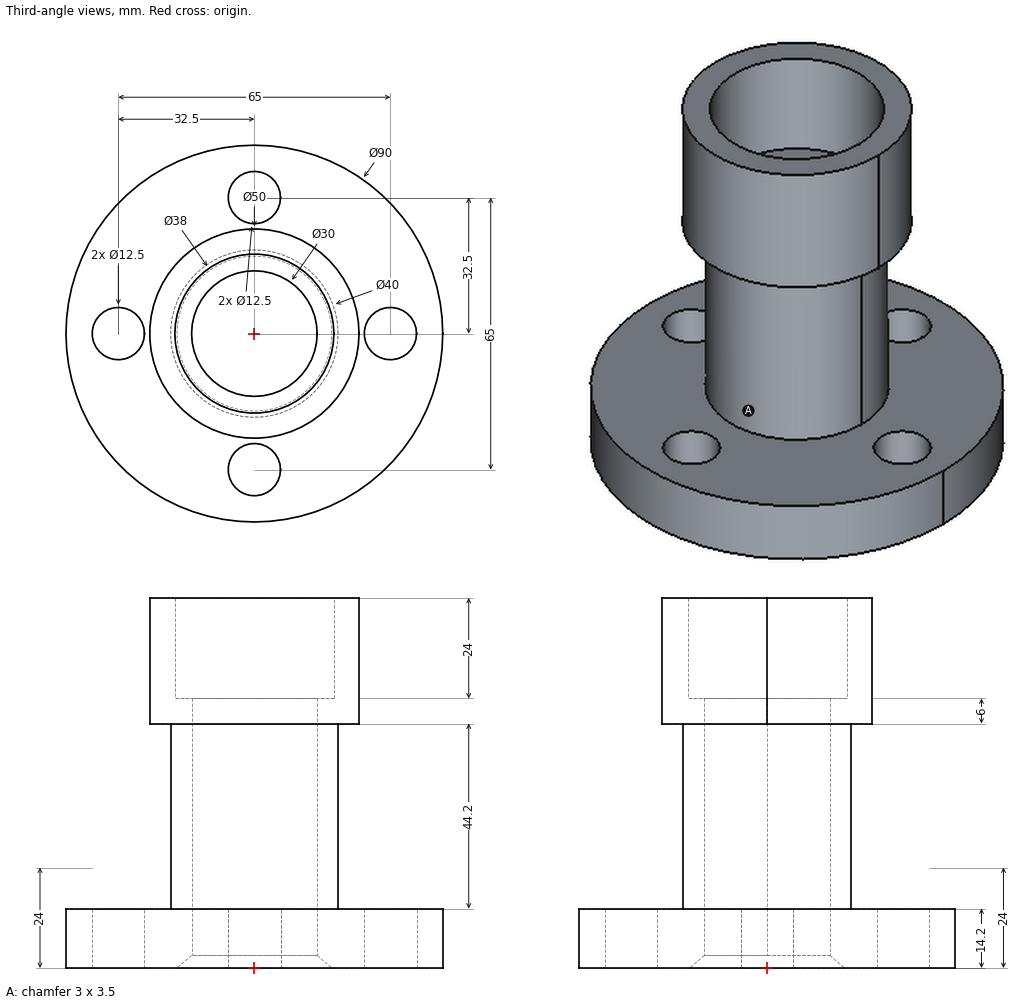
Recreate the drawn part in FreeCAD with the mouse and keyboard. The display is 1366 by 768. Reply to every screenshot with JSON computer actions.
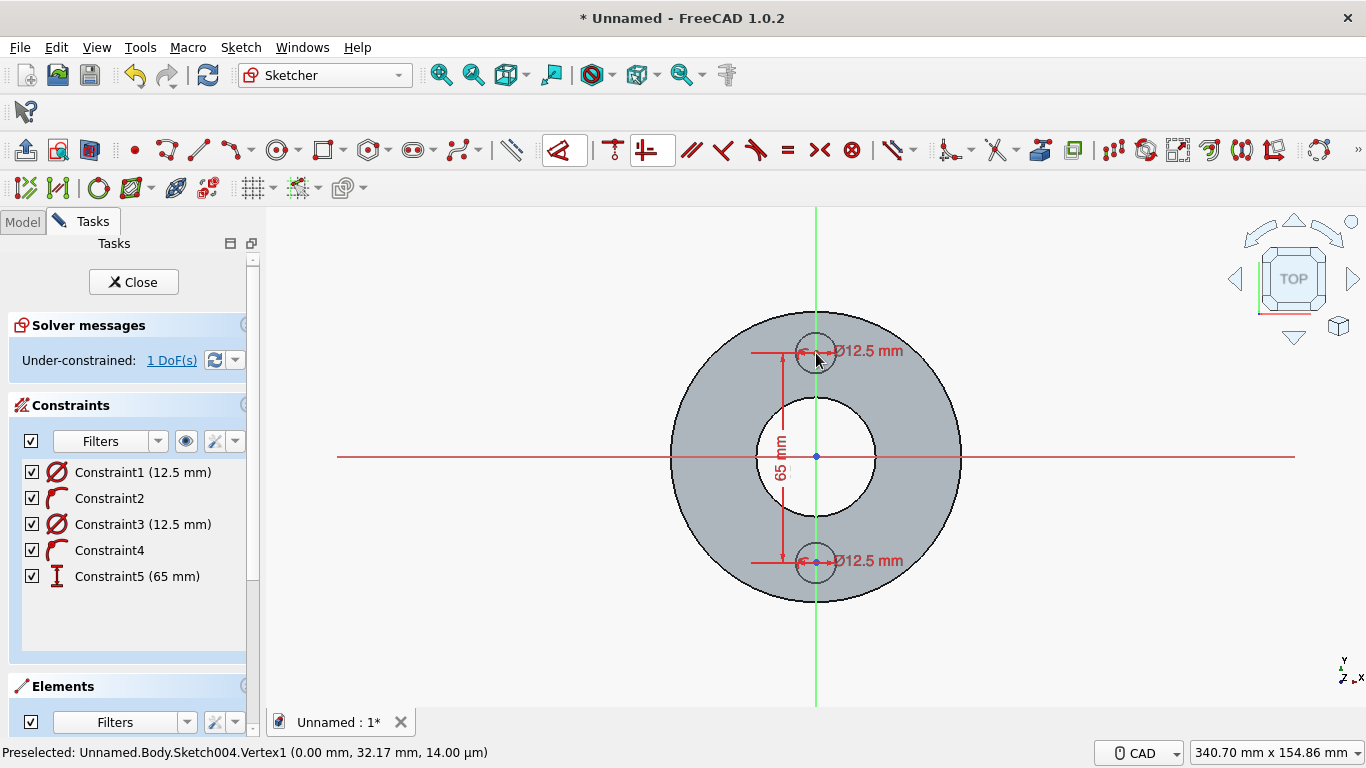
{"action": "left_click", "coordinate": [582, 150]}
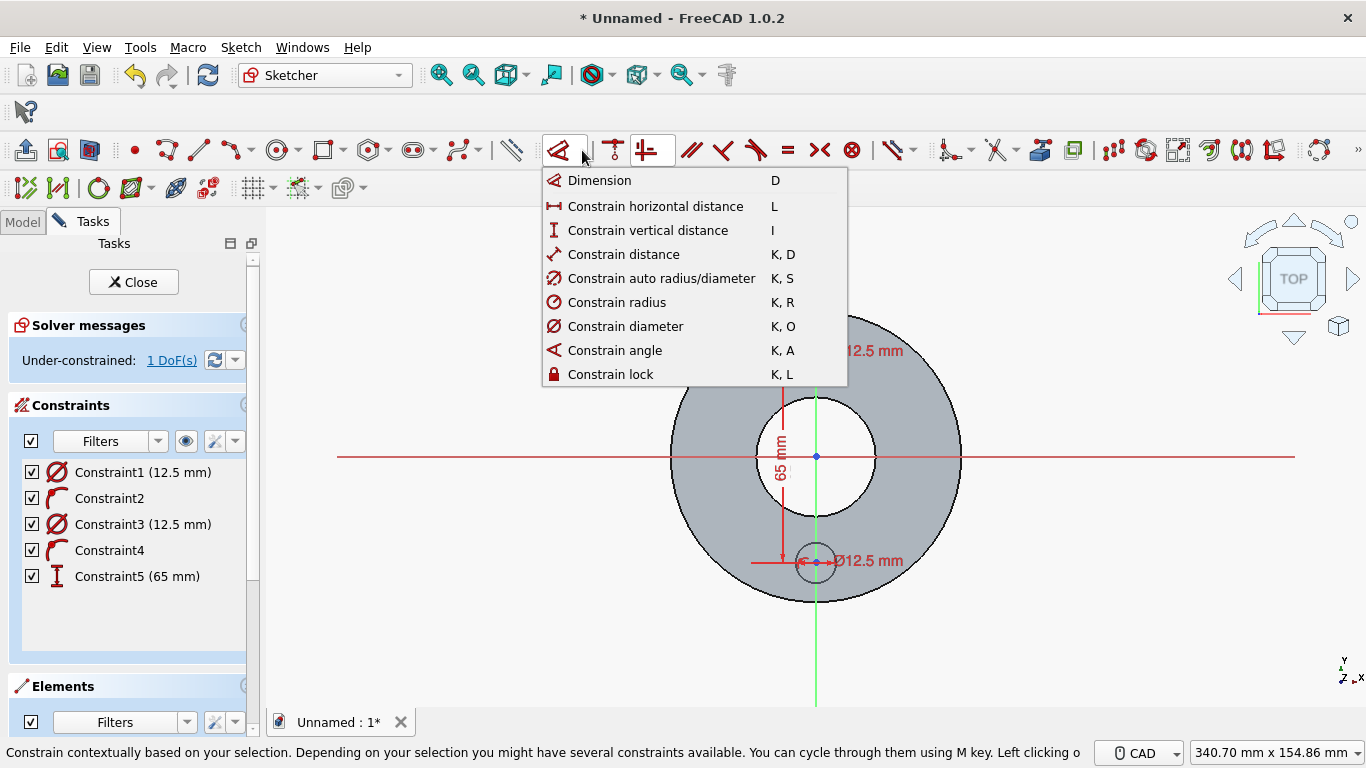
{"action": "left_click", "coordinate": [695, 230]}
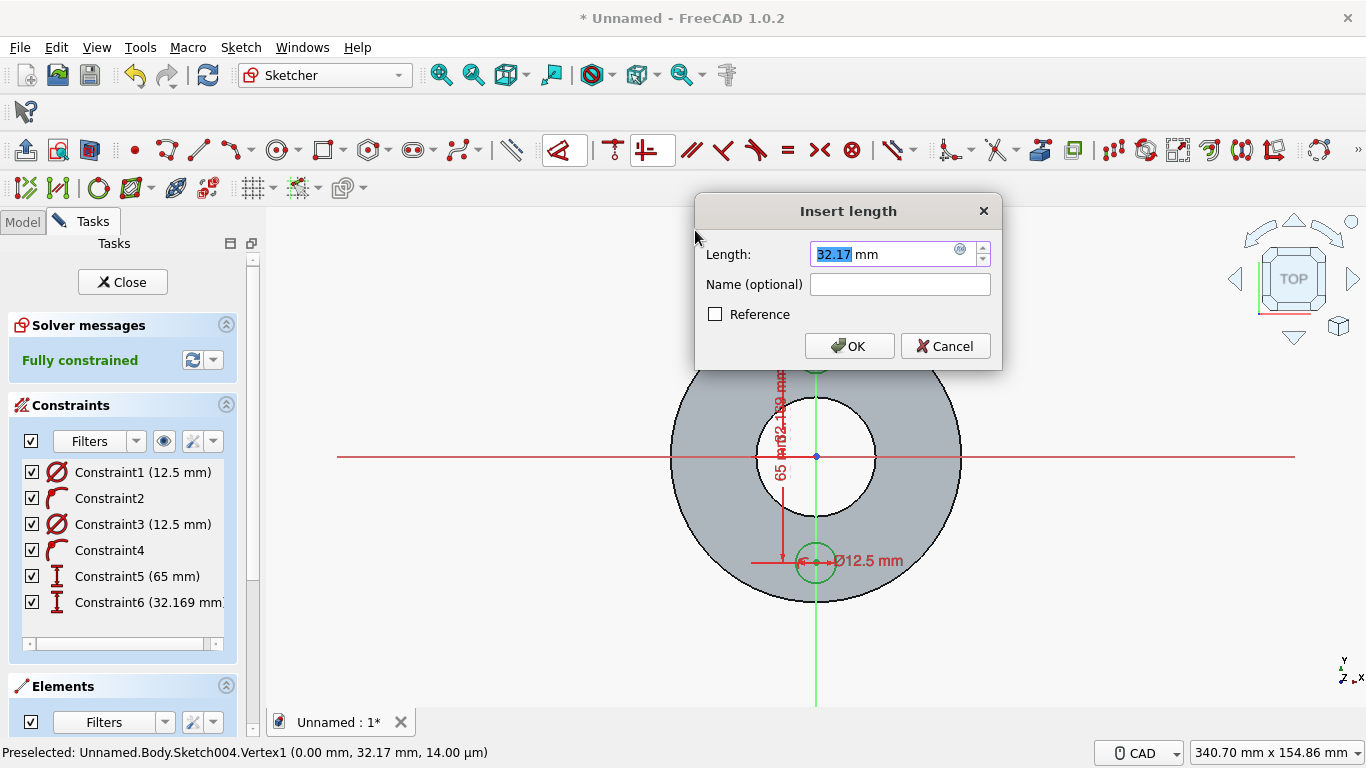
{"action": "type", "text": "32.5"}
{"action": "key", "text": "Return"}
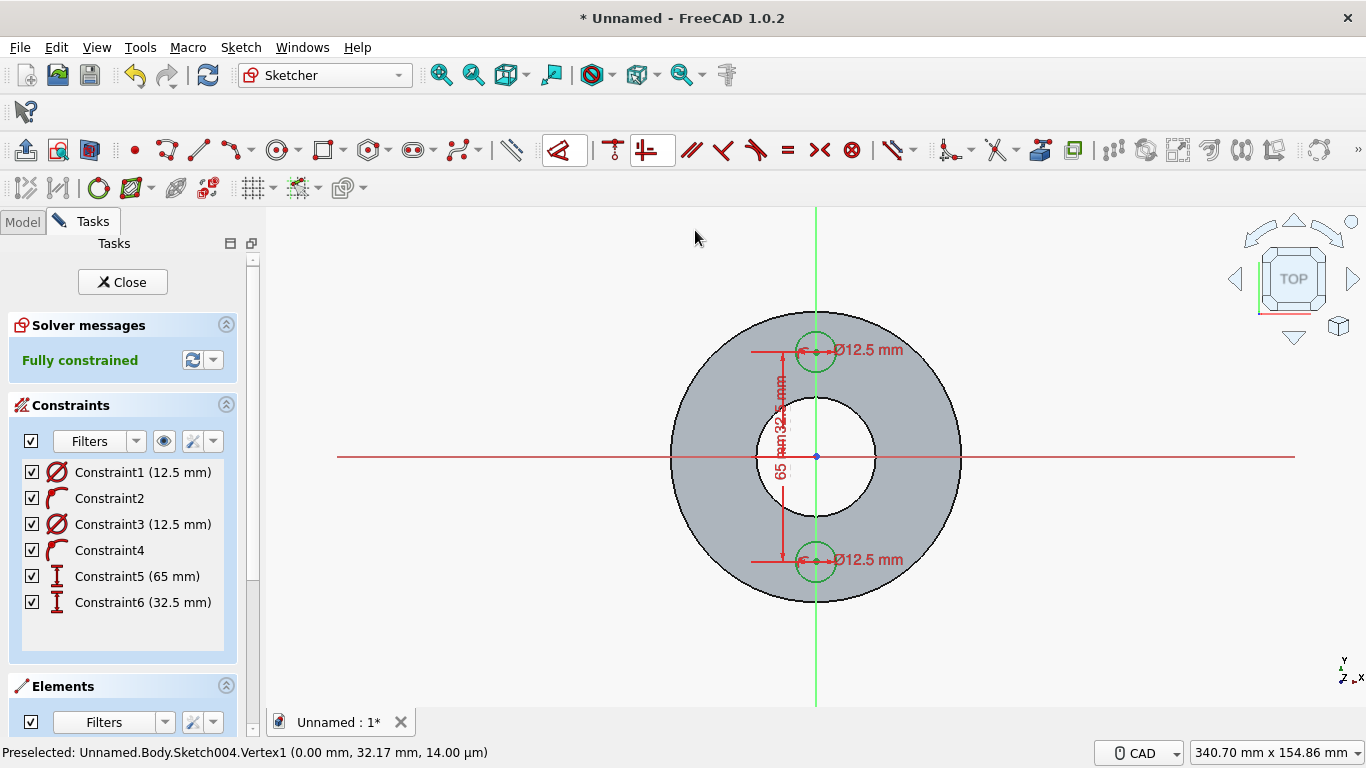
{"action": "left_click", "coordinate": [123, 282]}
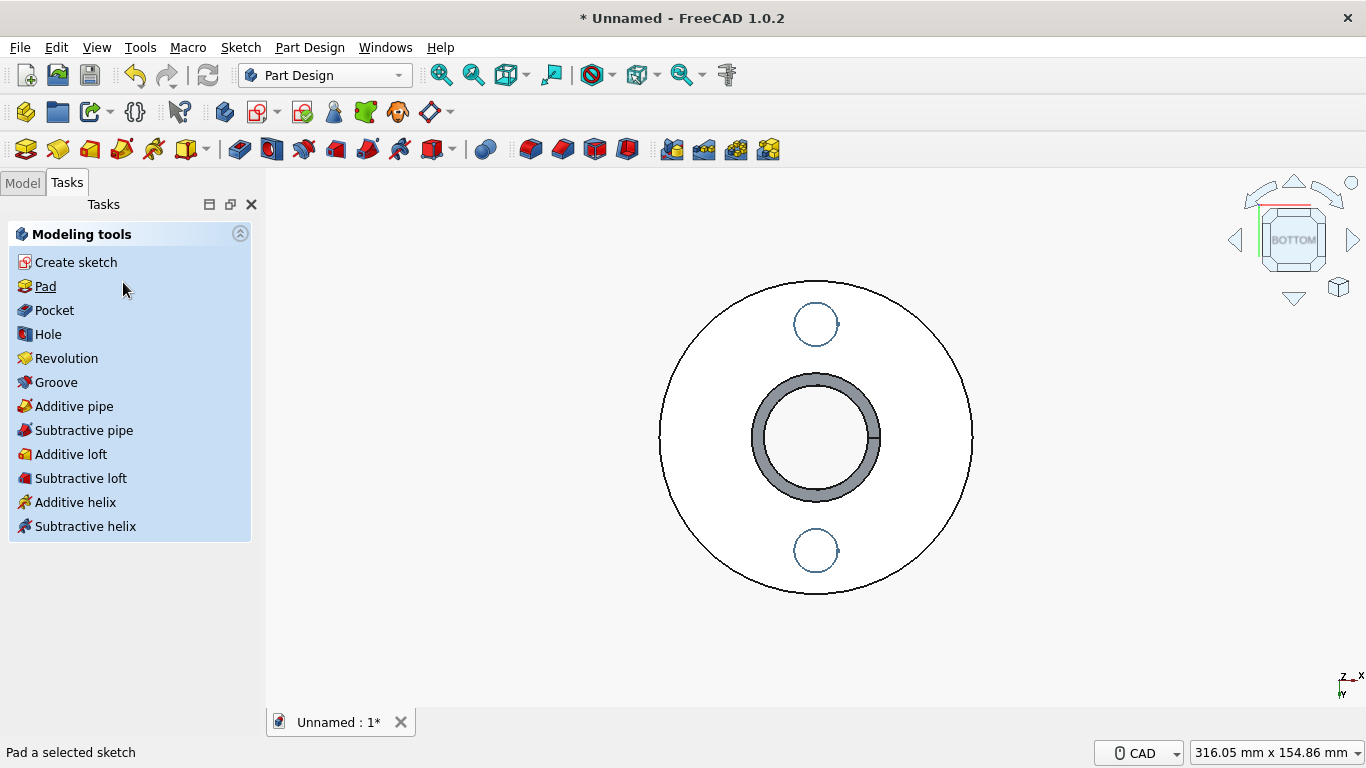
{"action": "left_click", "coordinate": [240, 150]}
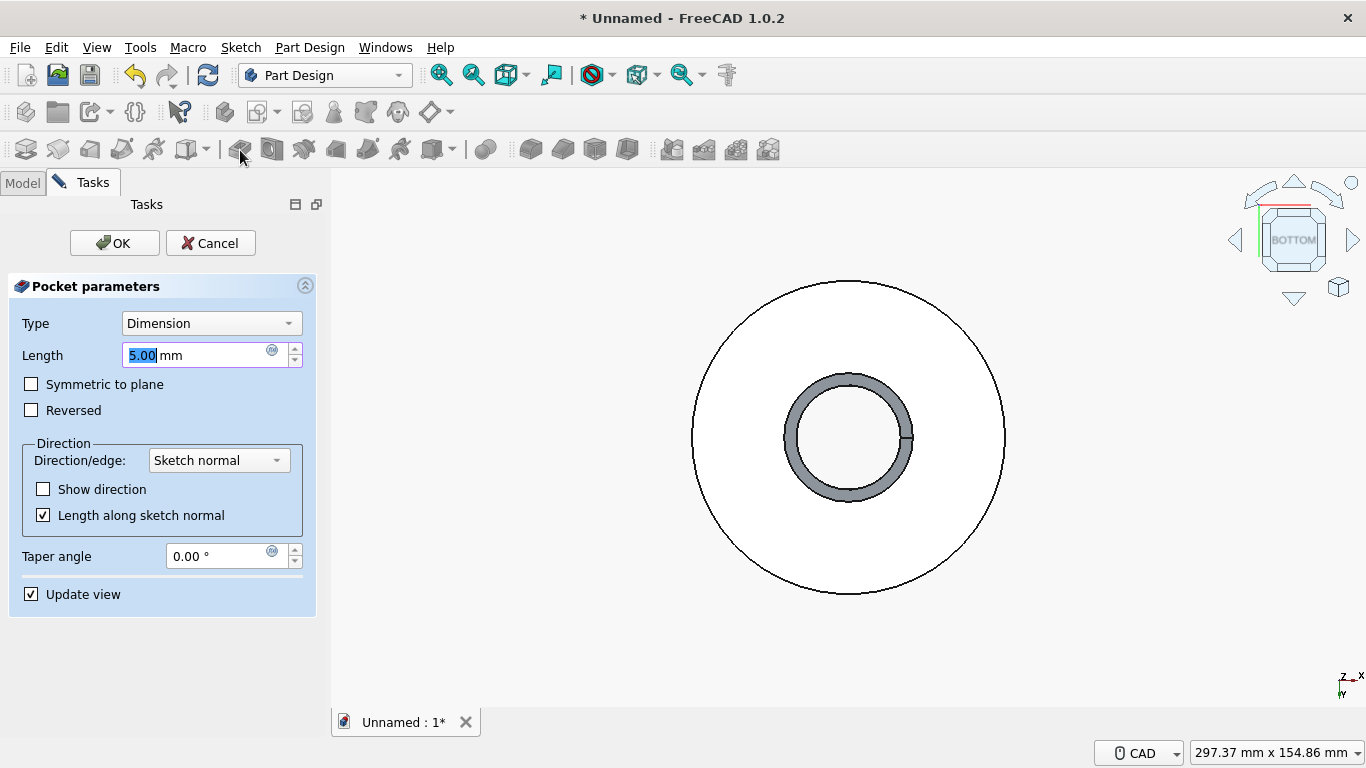
{"action": "type", "text": "24"}
{"action": "key", "text": "Tab"}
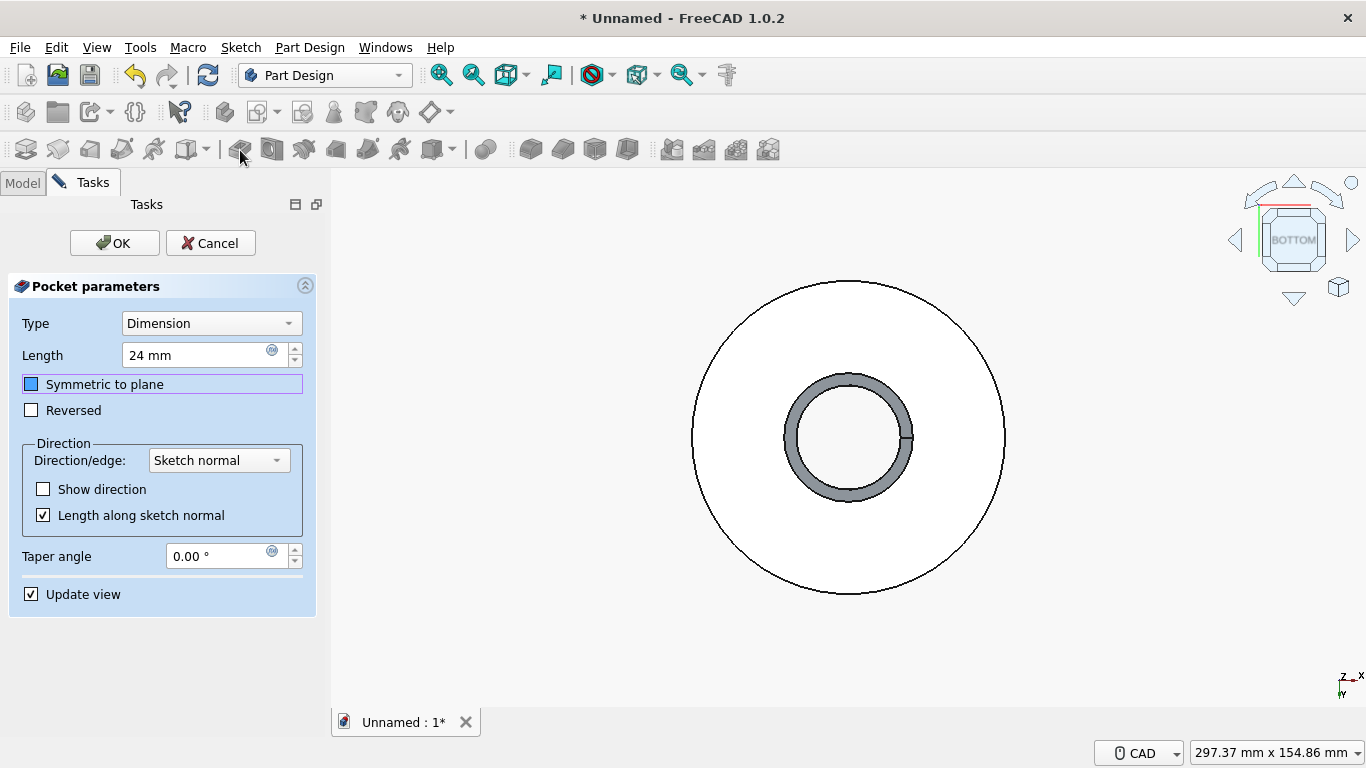
{"action": "left_click", "coordinate": [30, 410]}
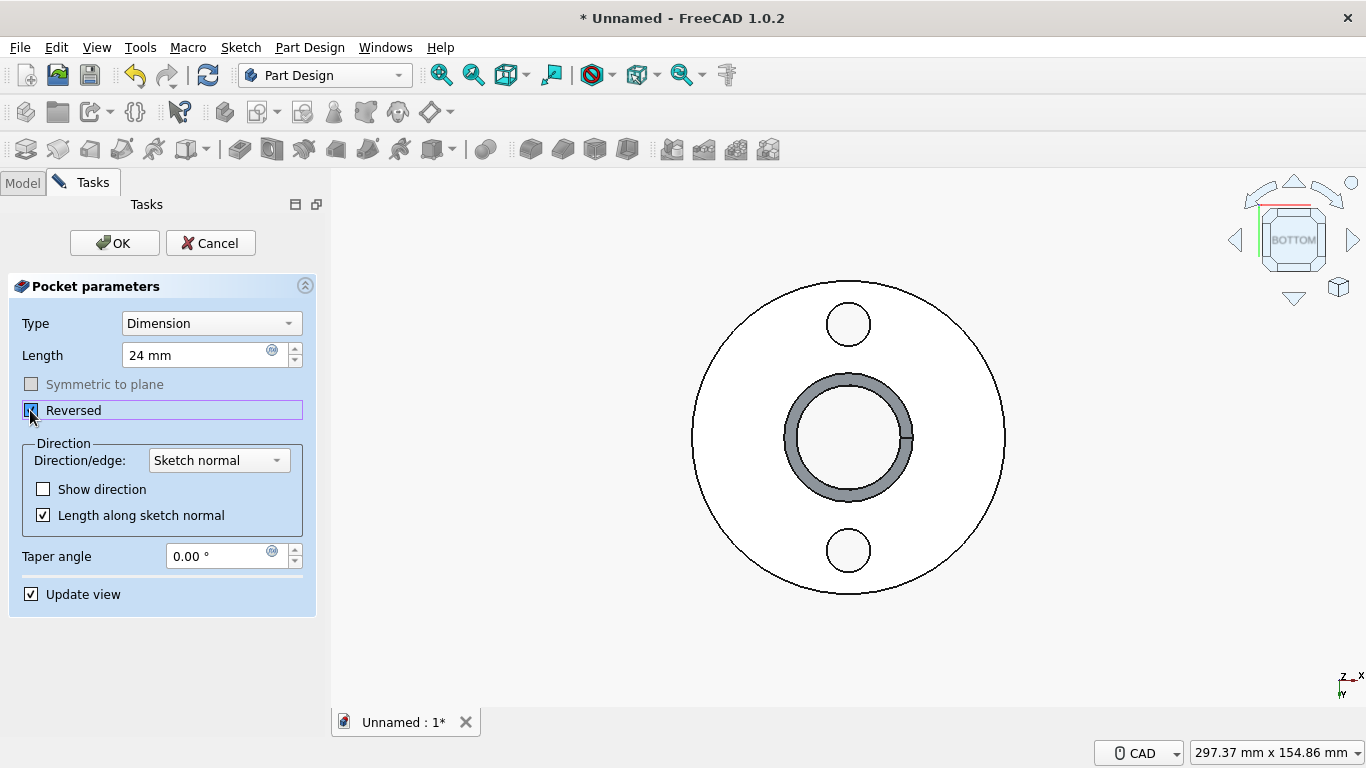
{"action": "left_click", "coordinate": [115, 243]}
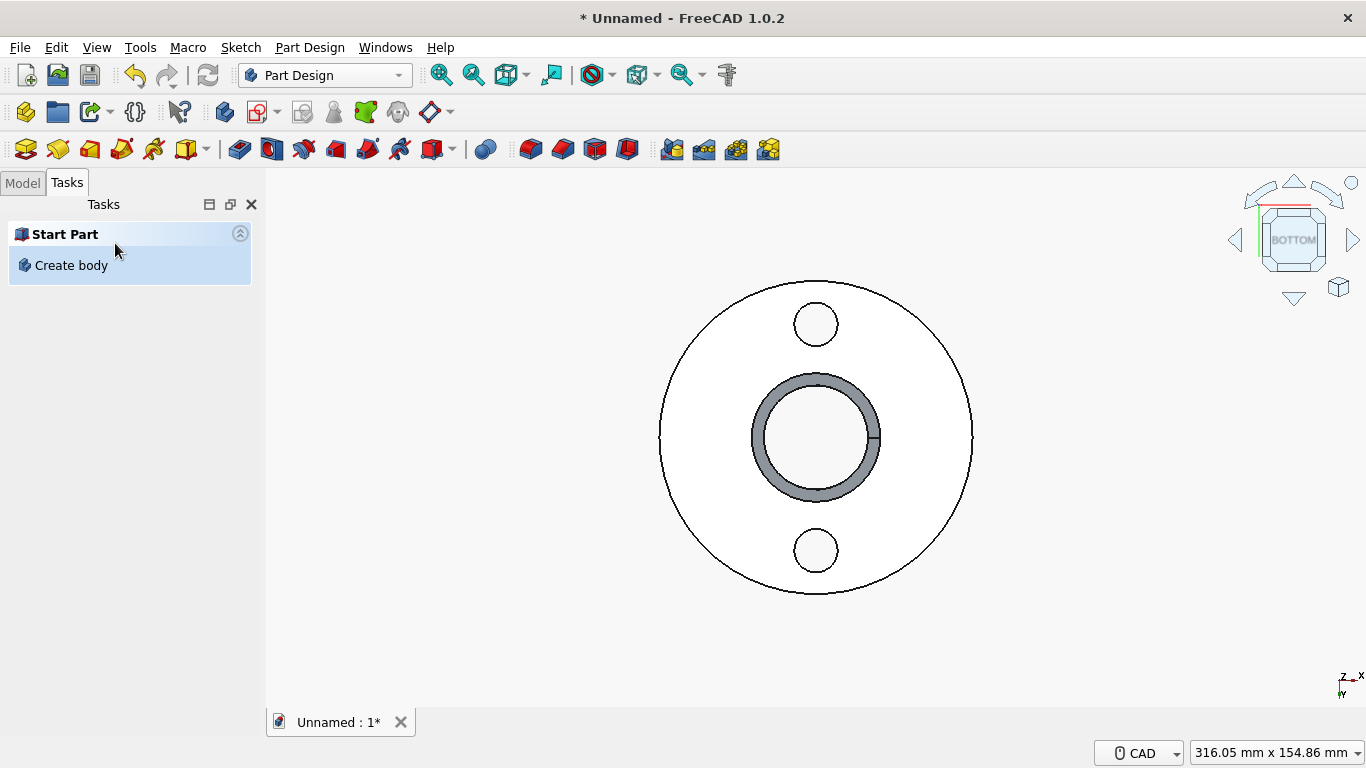
{"action": "left_click", "coordinate": [727, 481]}